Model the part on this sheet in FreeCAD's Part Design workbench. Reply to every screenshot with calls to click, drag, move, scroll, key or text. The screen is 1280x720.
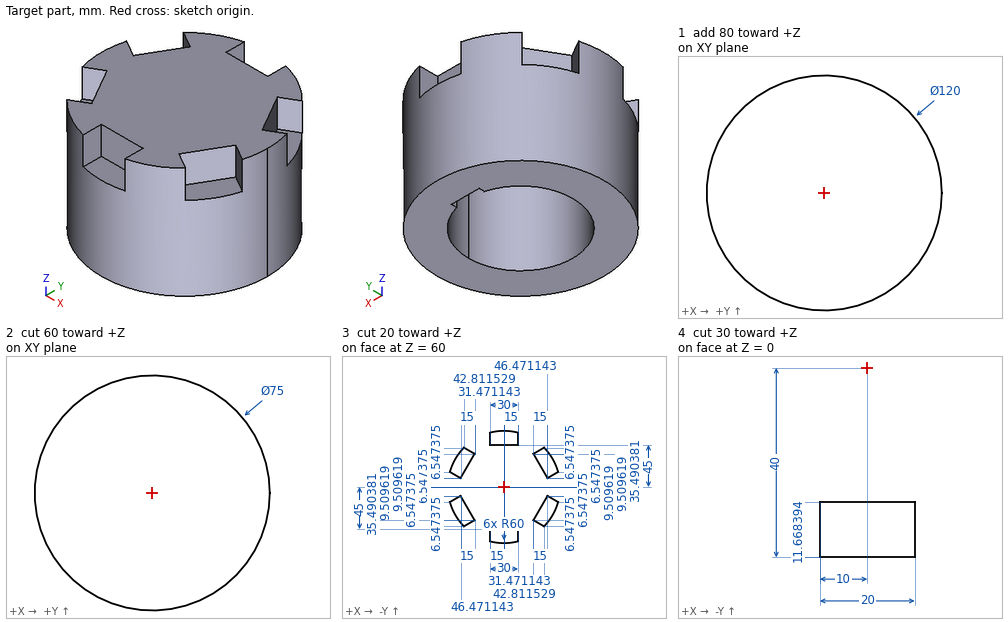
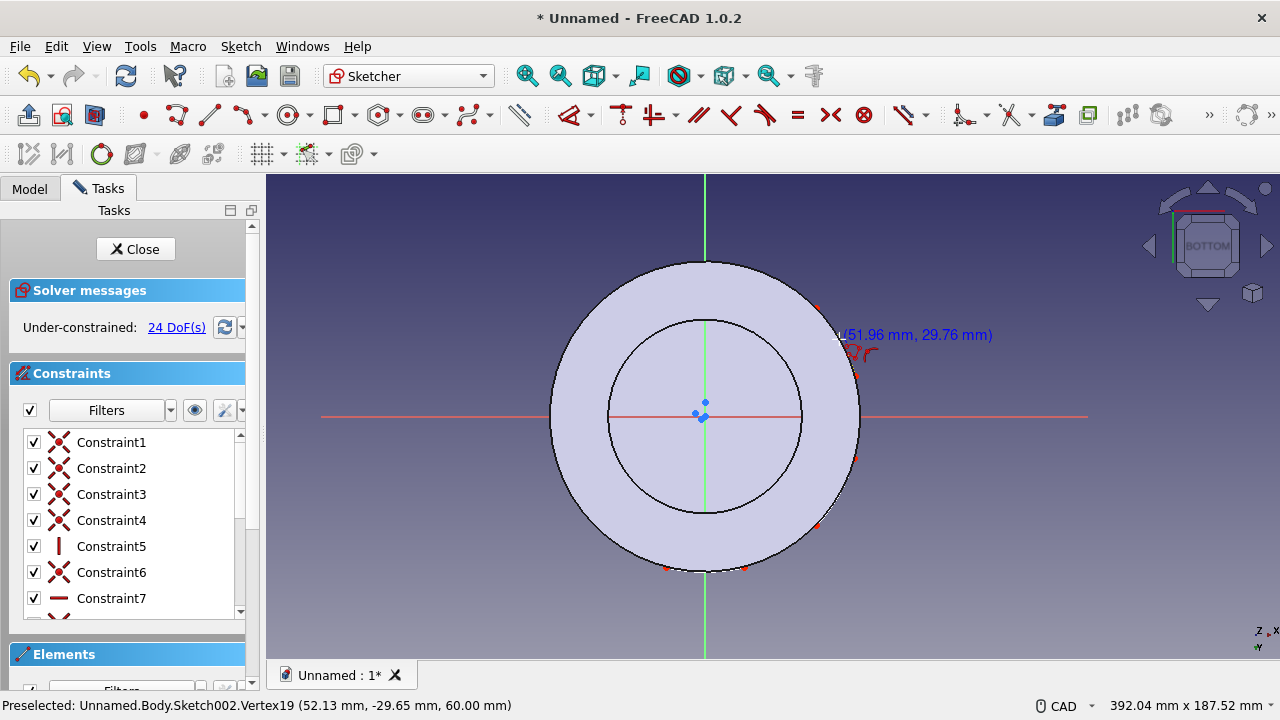
click(744, 266)
click(744, 300)
click(666, 300)
click(666, 266)
right_click(666, 266)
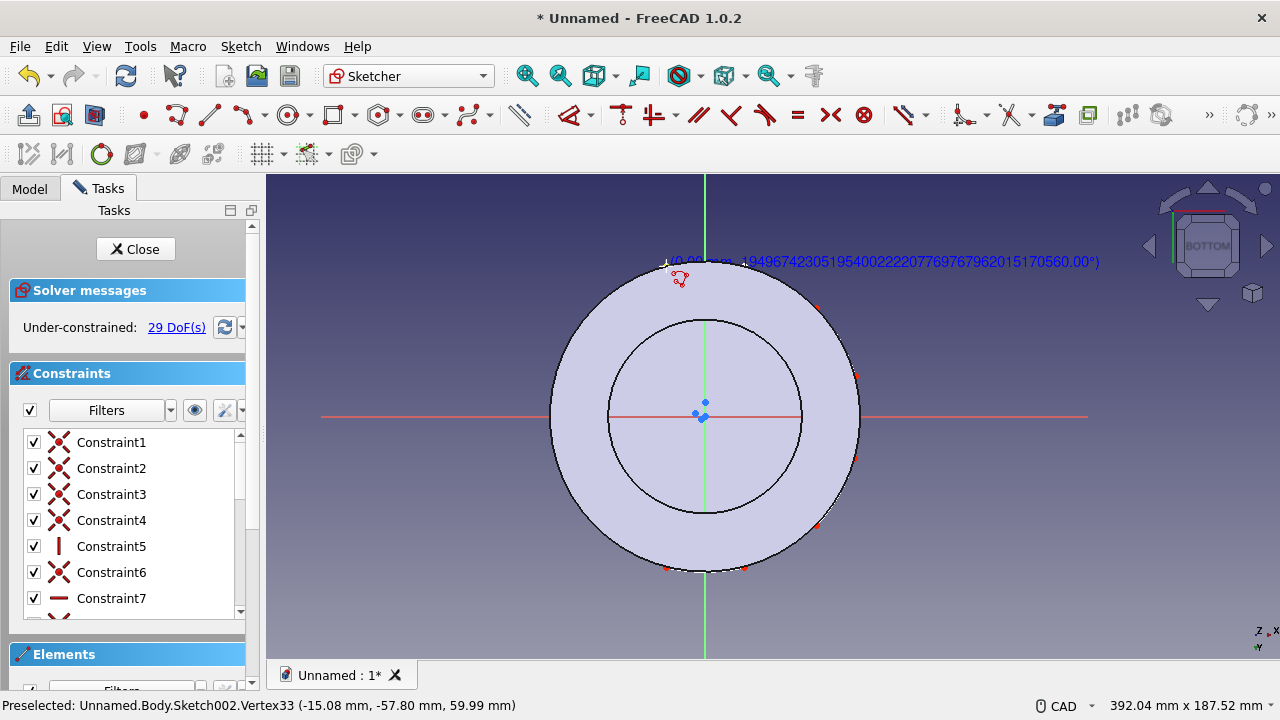
click(242, 116)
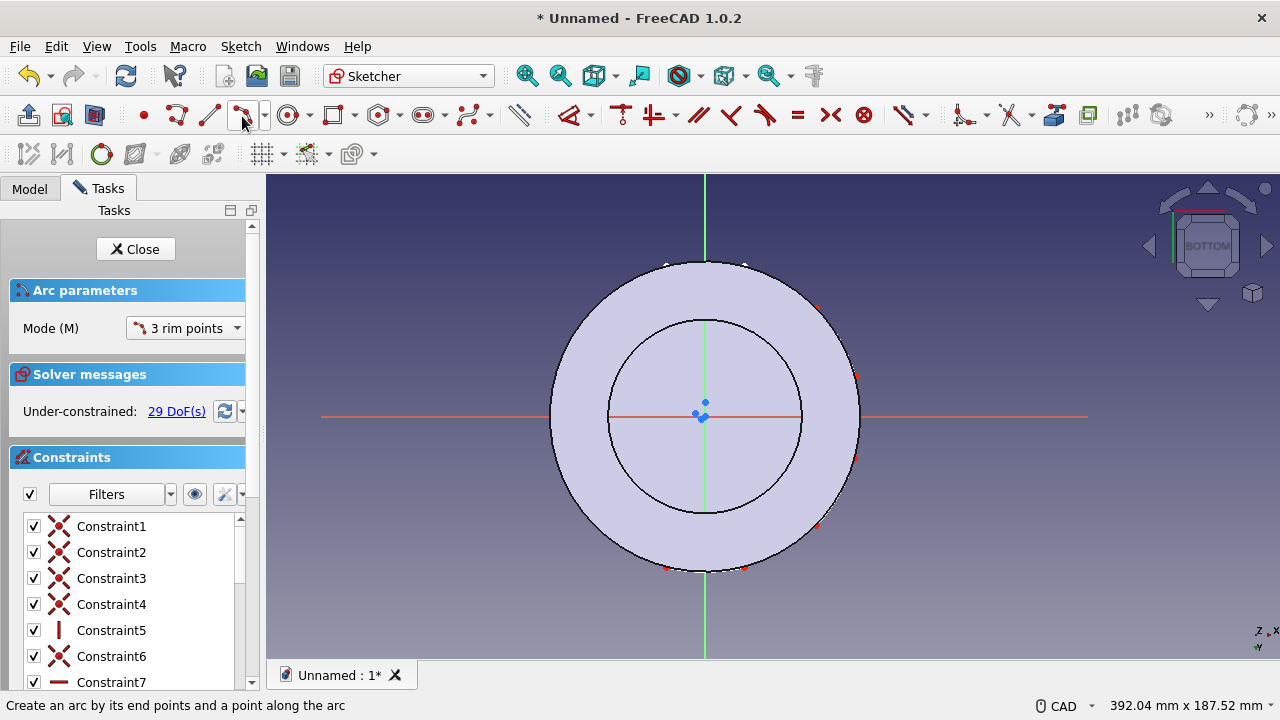
click(666, 267)
click(744, 267)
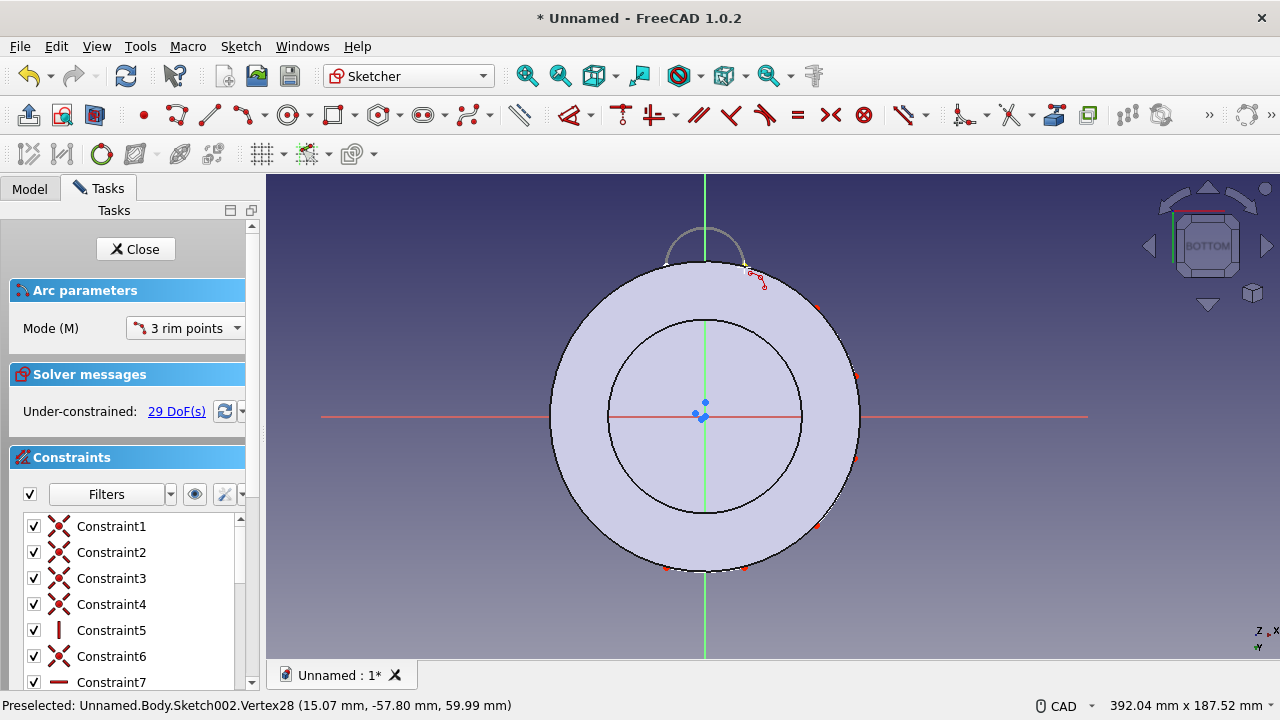
scroll(713, 262, up, 7)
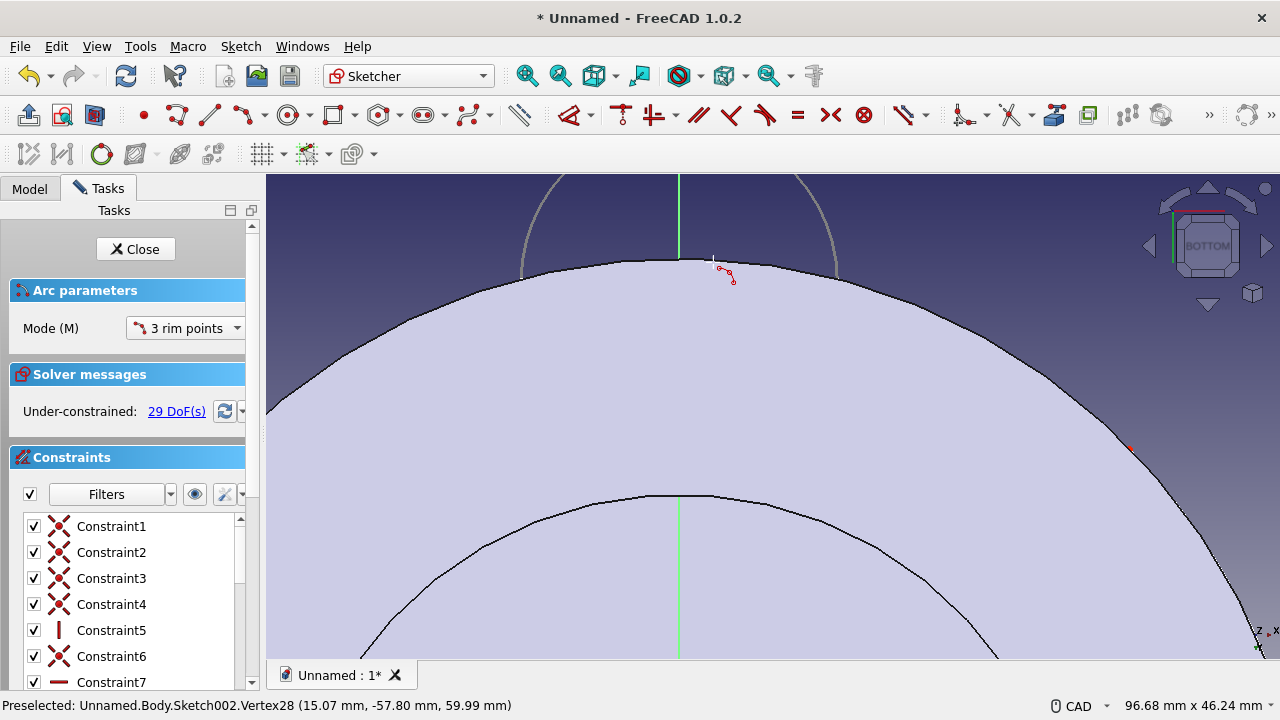
click(711, 259)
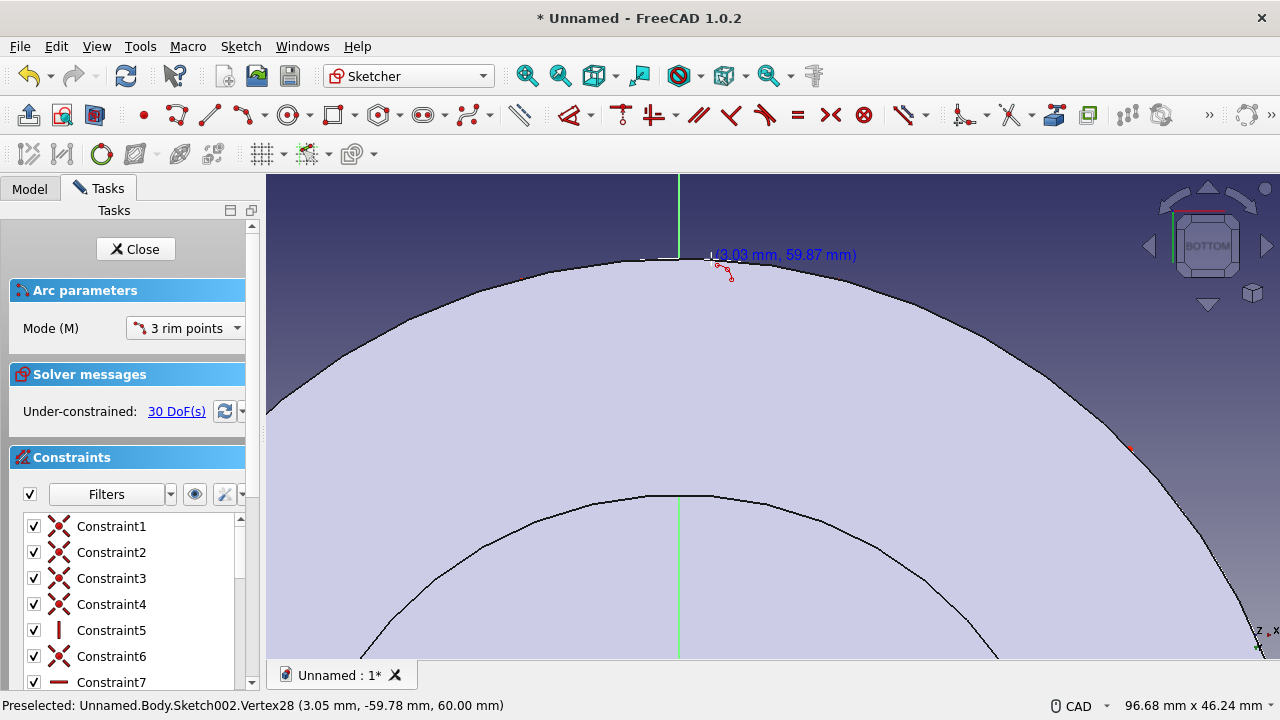
click(177, 116)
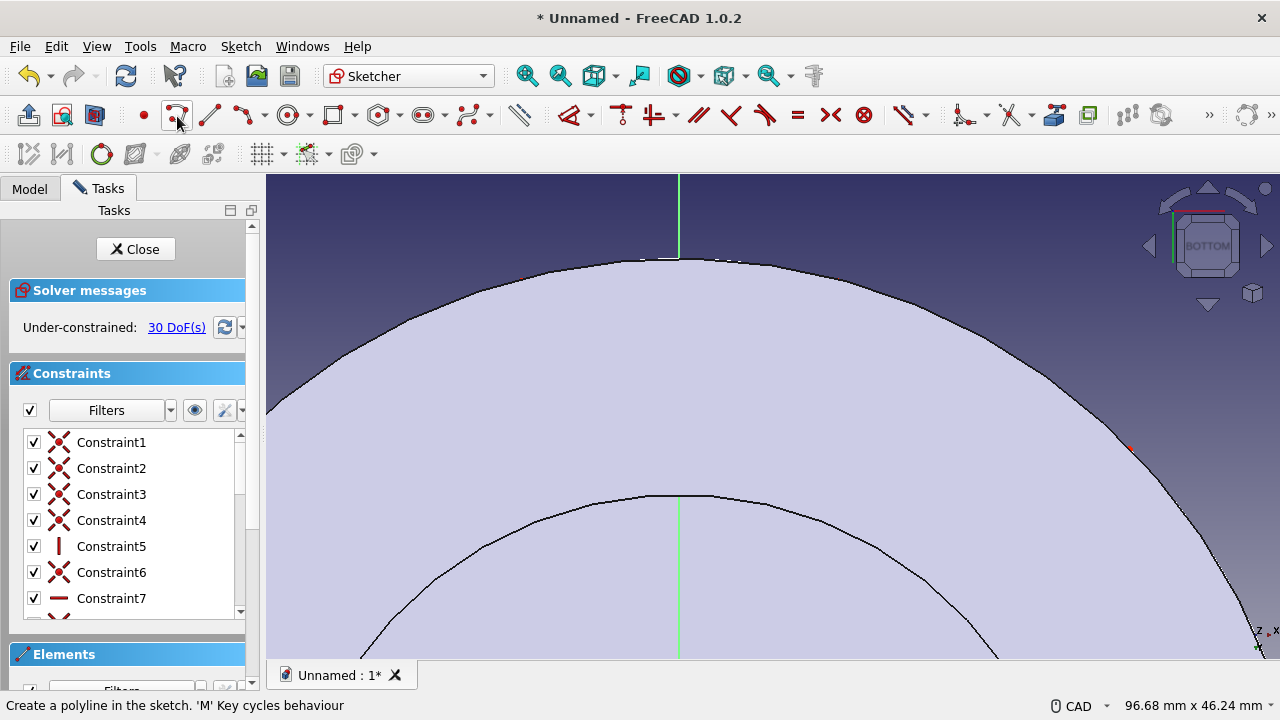
scroll(713, 262, down, 7)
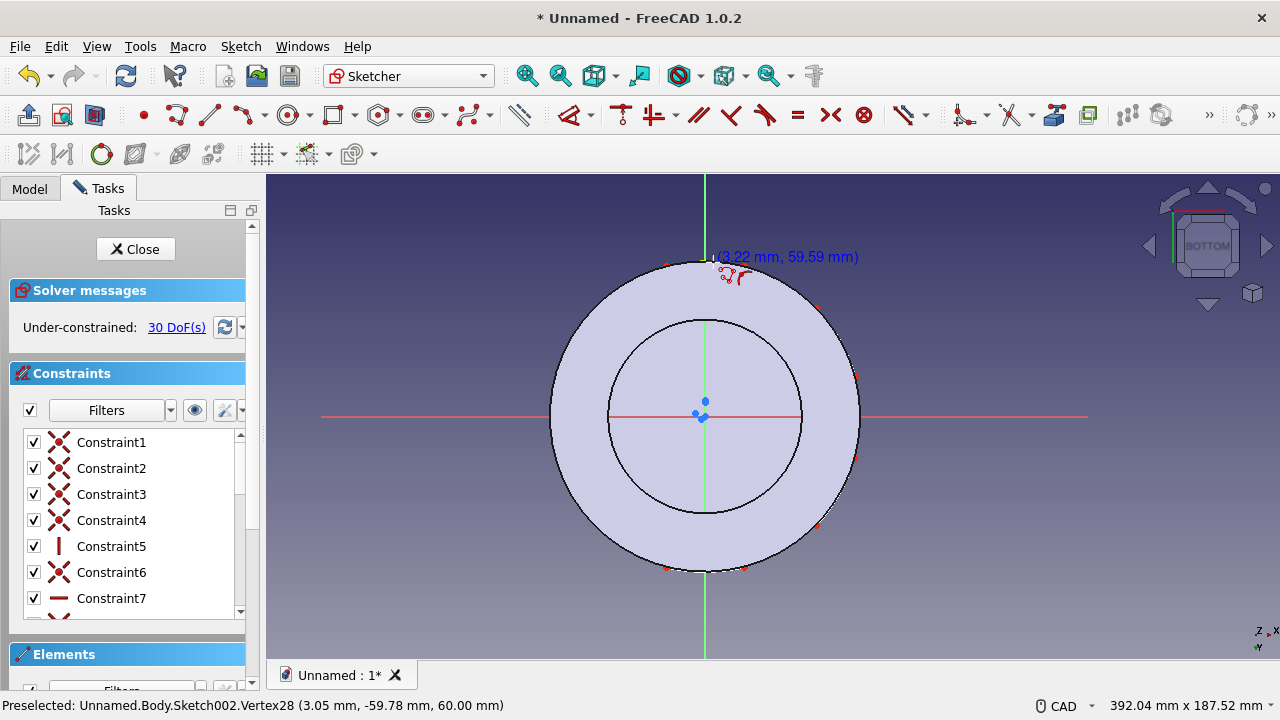
click(594, 308)
click(624, 325)
click(585, 392)
click(555, 375)
right_click(555, 375)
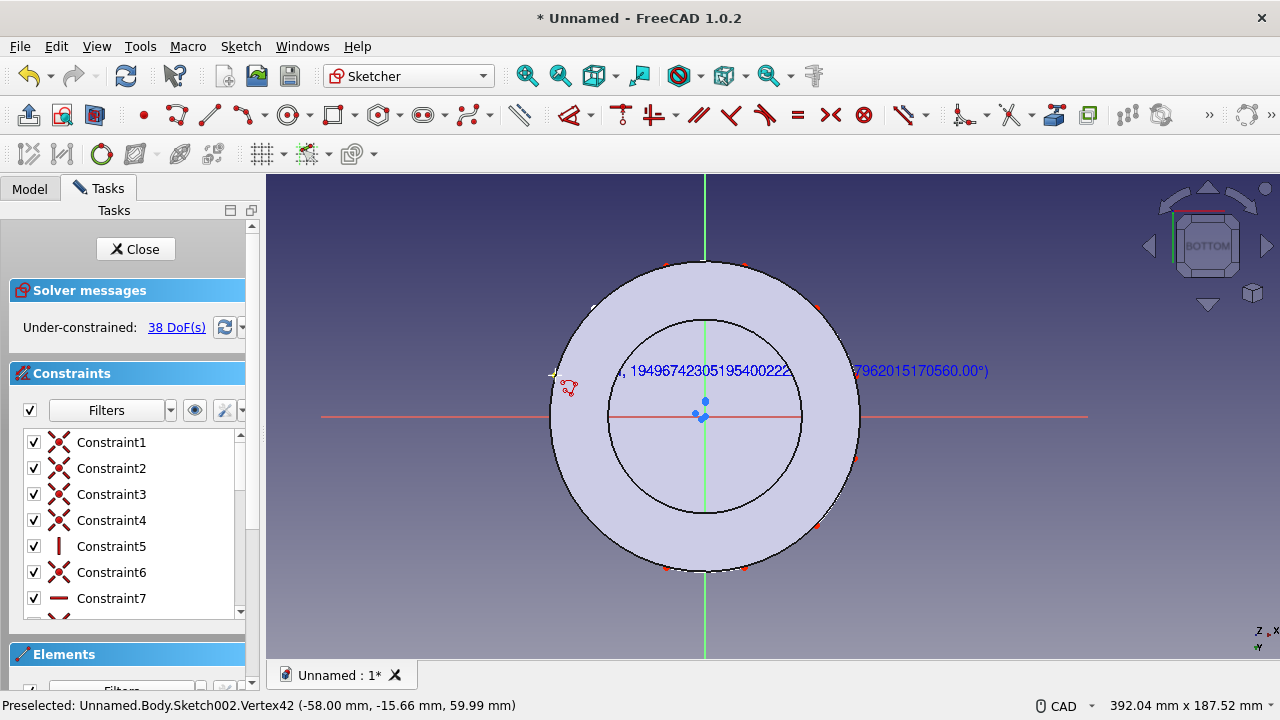
click(242, 116)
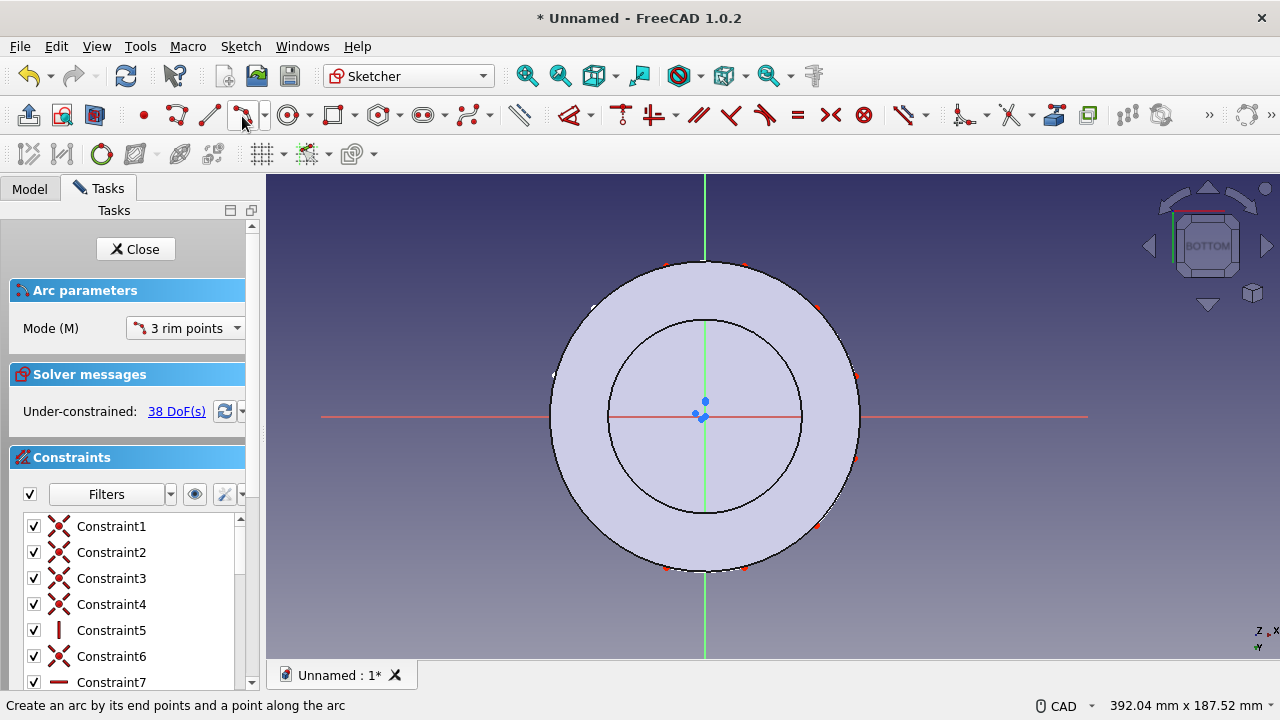
click(555, 376)
click(594, 309)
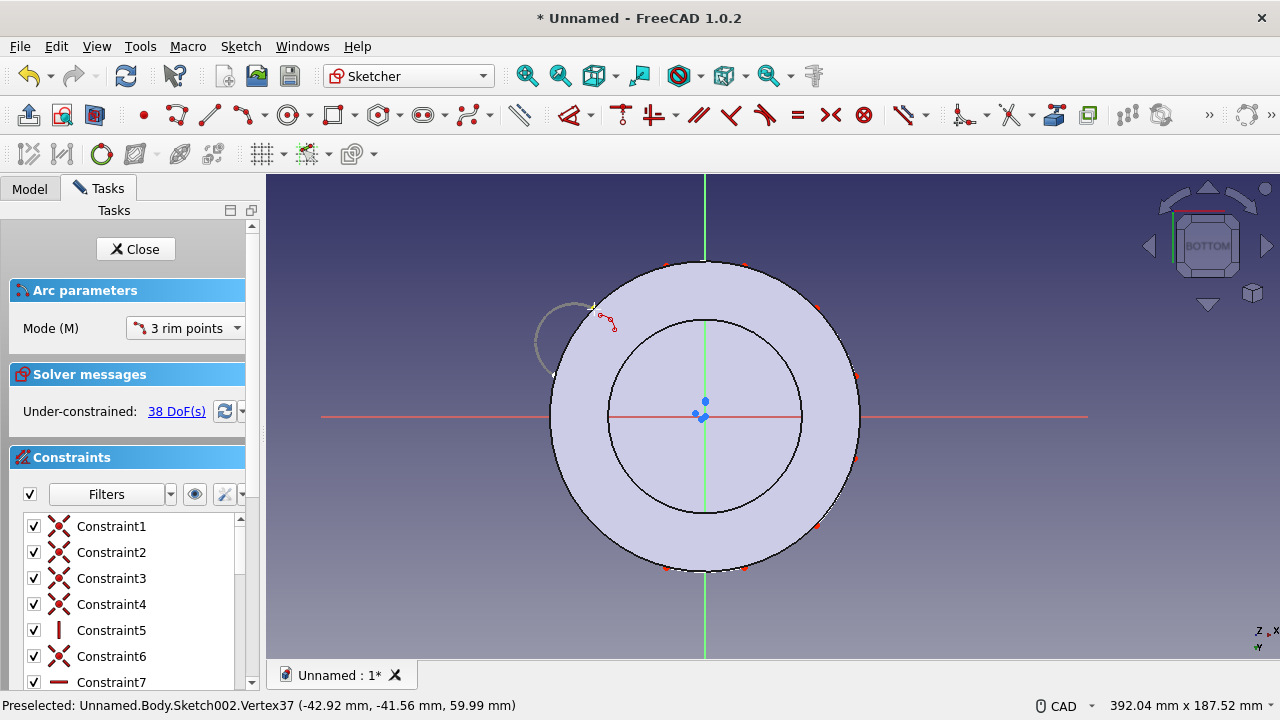
scroll(571, 339, up, 6)